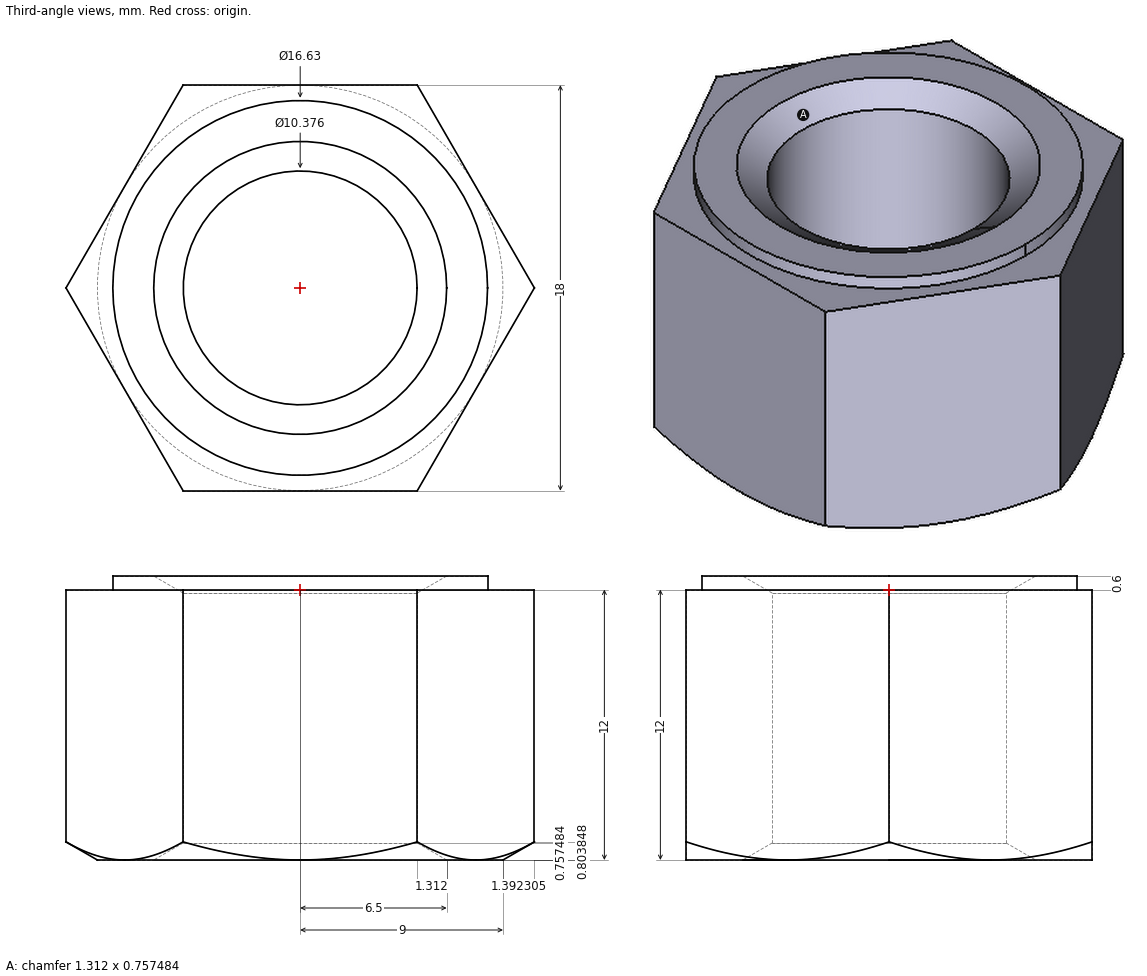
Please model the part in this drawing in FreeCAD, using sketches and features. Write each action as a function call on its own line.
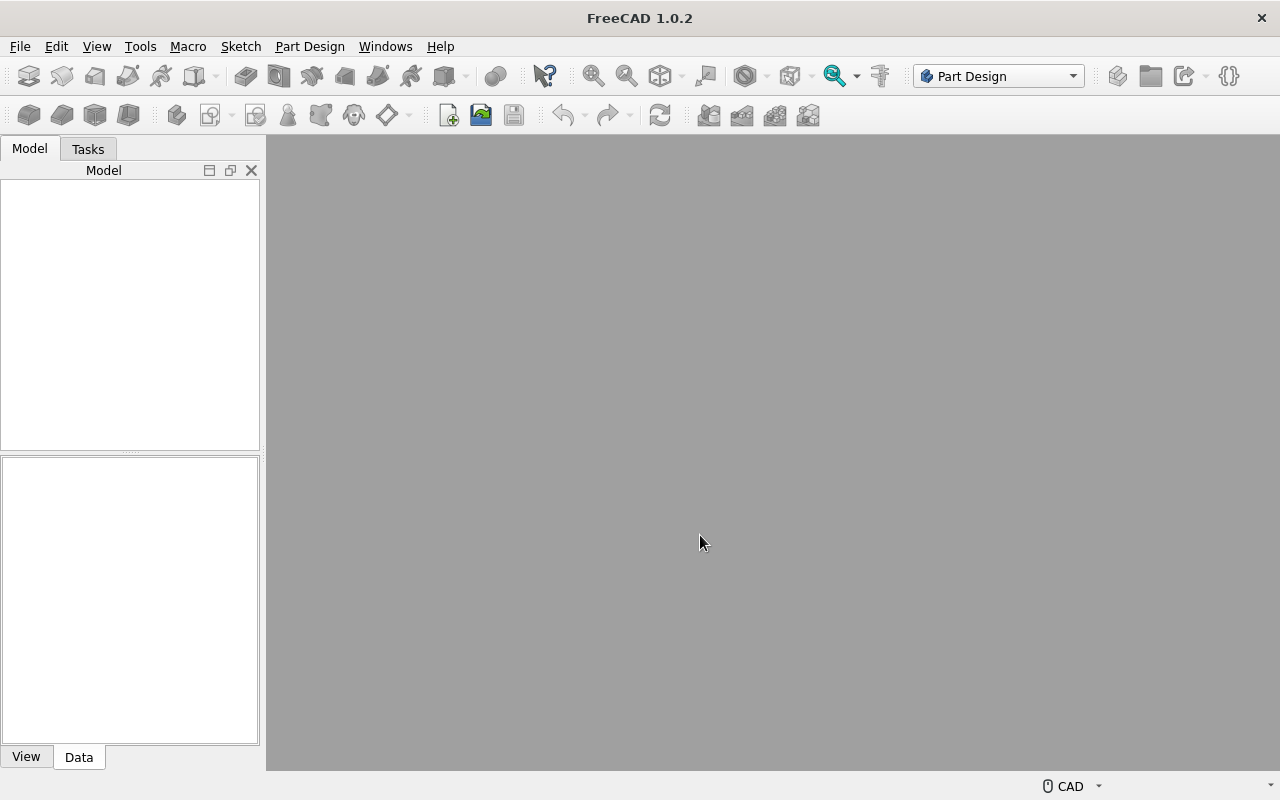
click(448, 116)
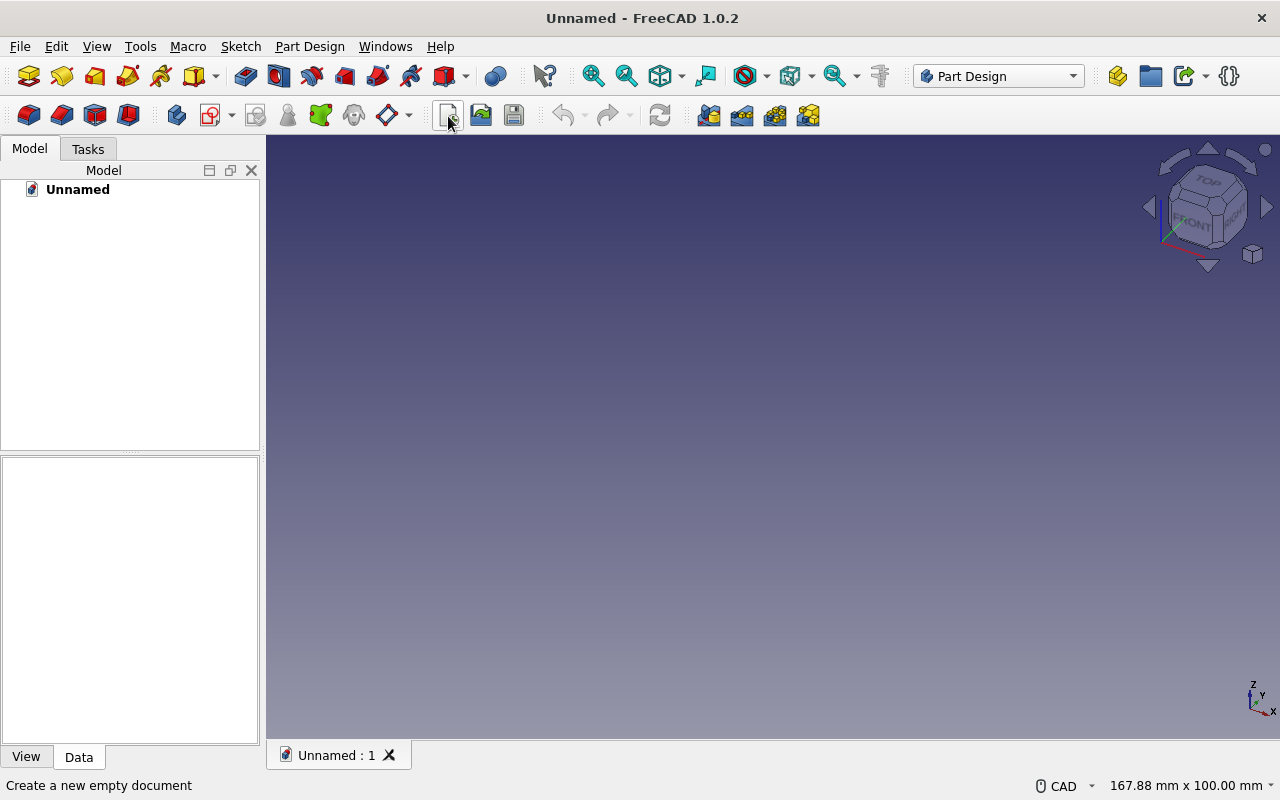
click(210, 116)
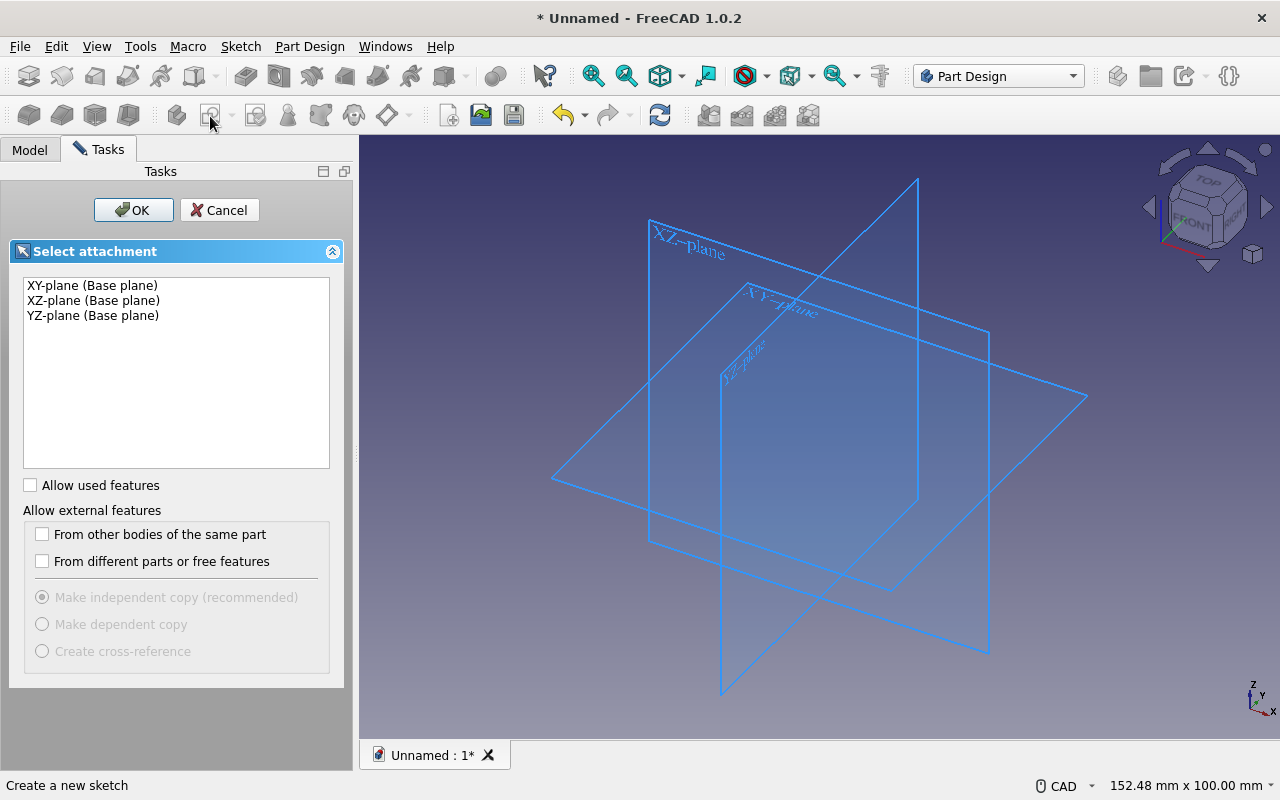
click(84, 286)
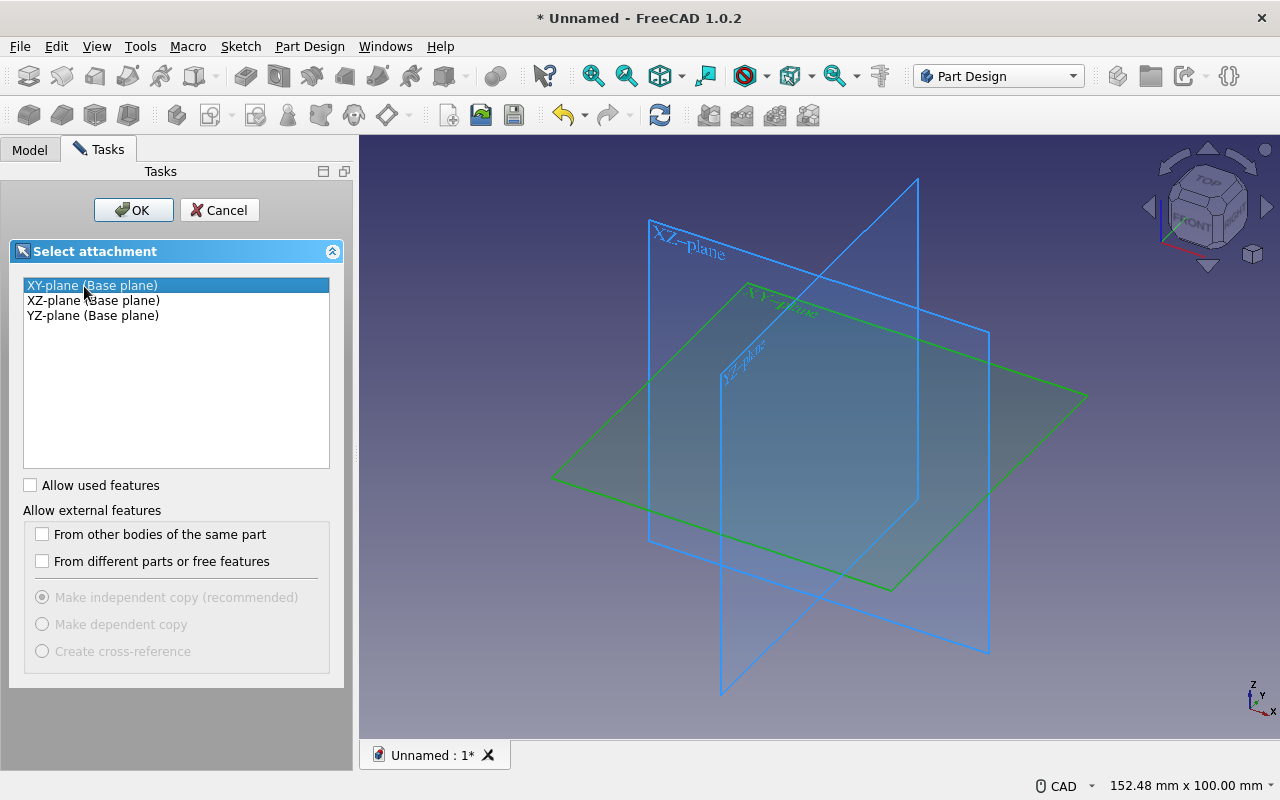
click(134, 210)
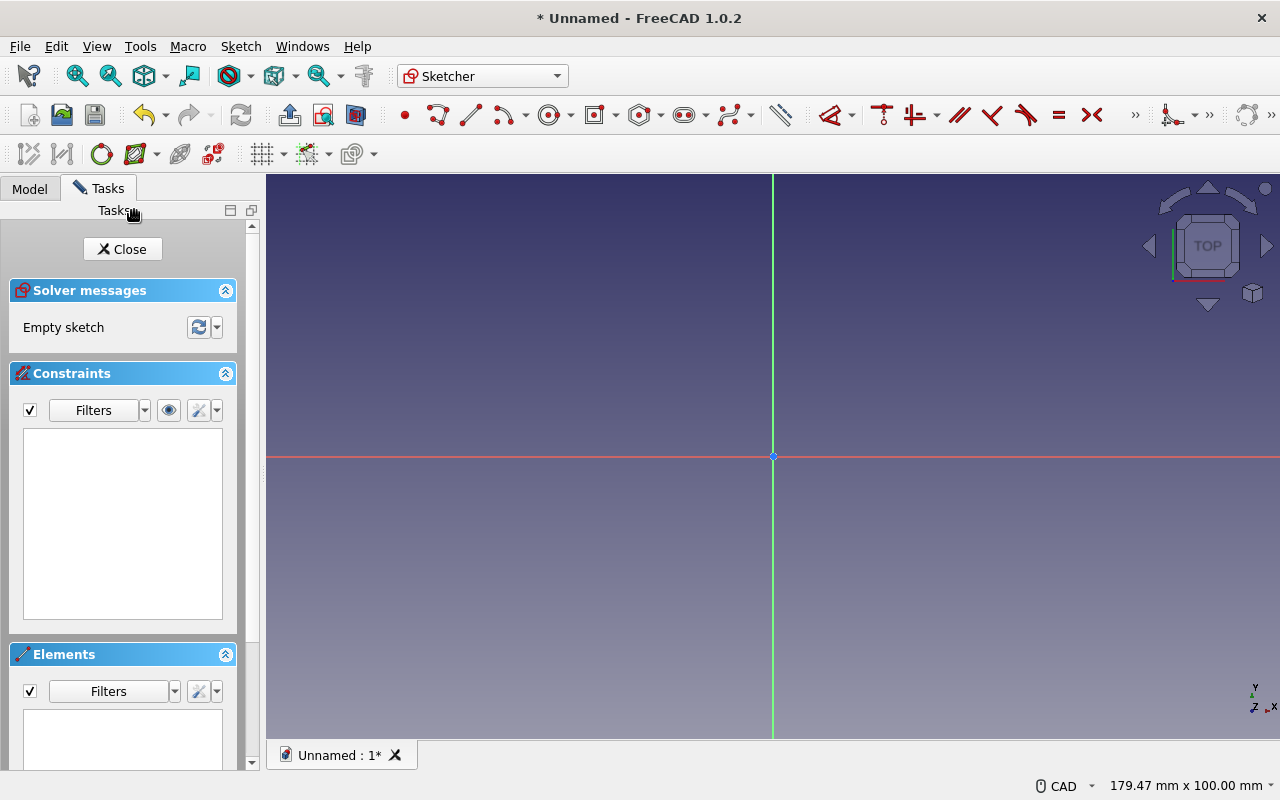
scroll(803, 456, up, 6)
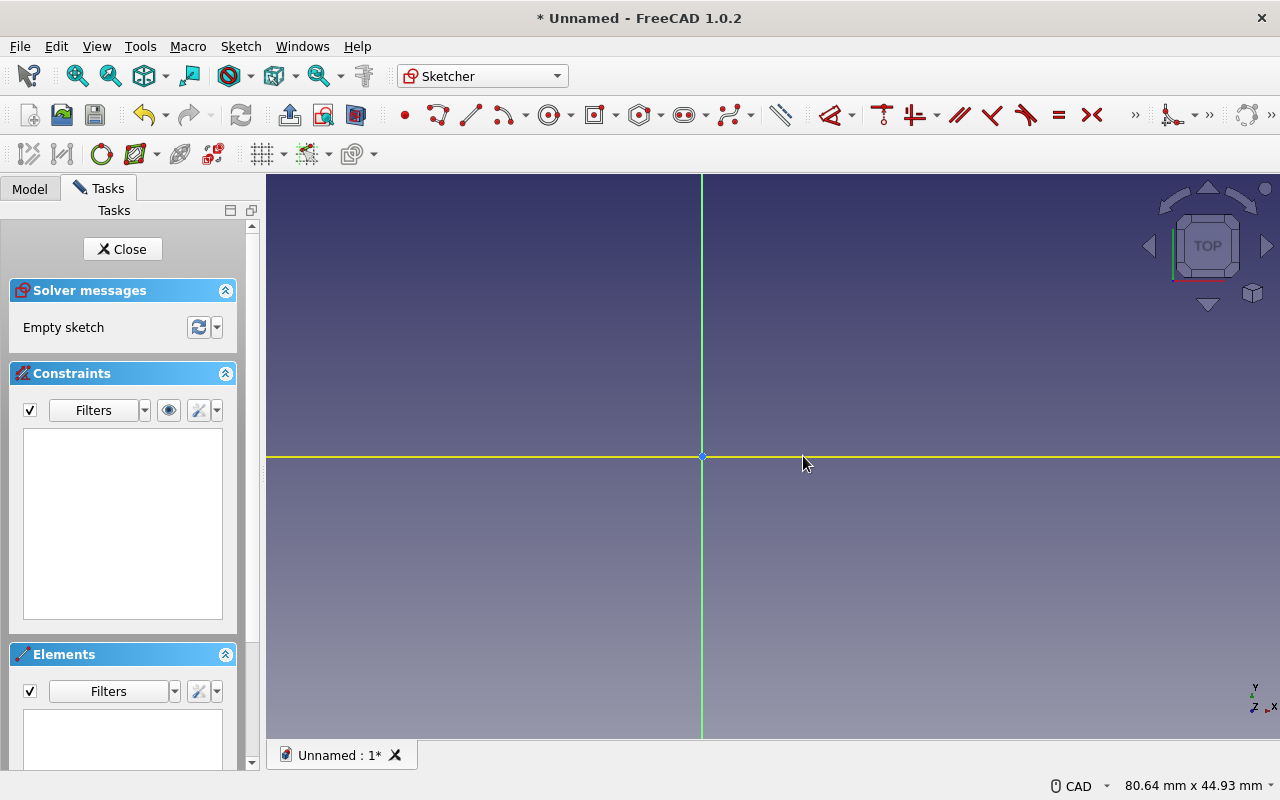
key(g)
key(p)
key(6)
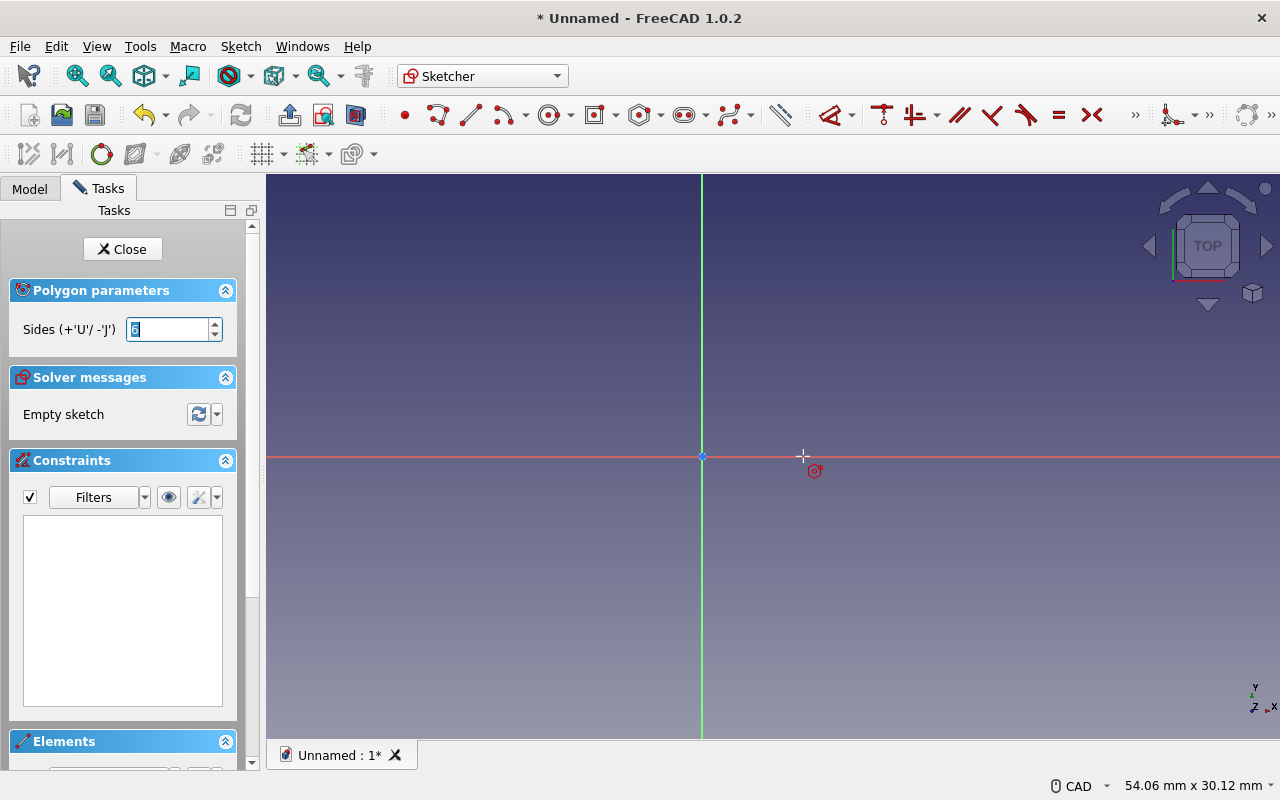
click(702, 456)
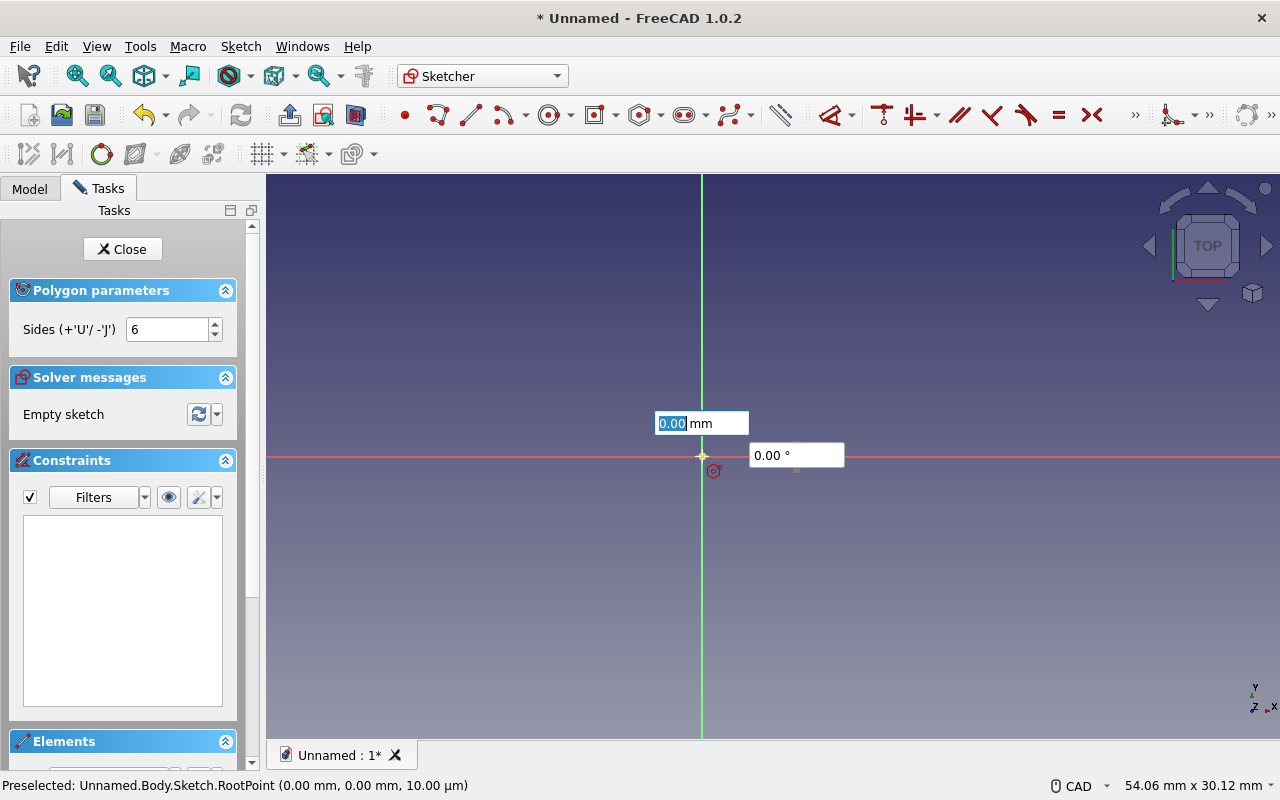
click(897, 456)
right_click(897, 456)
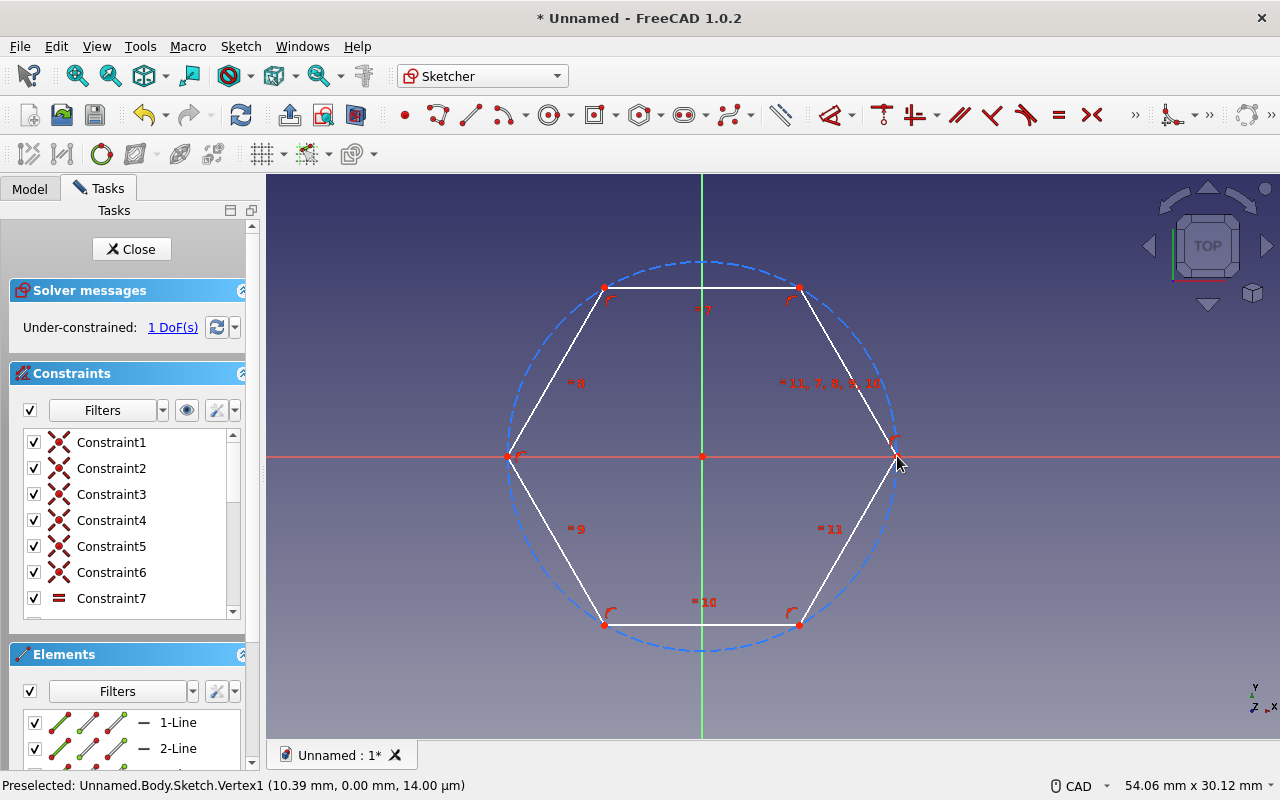
key(g)
key(c)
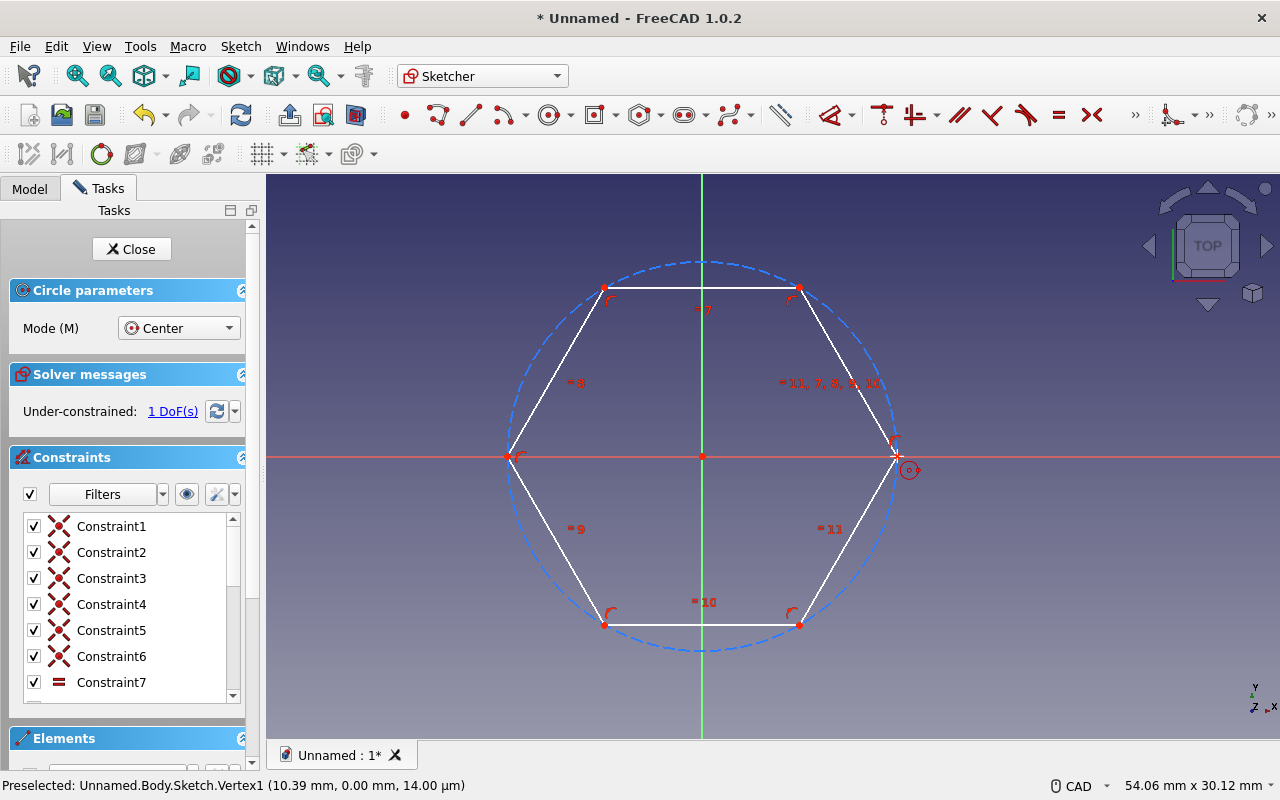
click(702, 456)
click(771, 388)
key(Escape)